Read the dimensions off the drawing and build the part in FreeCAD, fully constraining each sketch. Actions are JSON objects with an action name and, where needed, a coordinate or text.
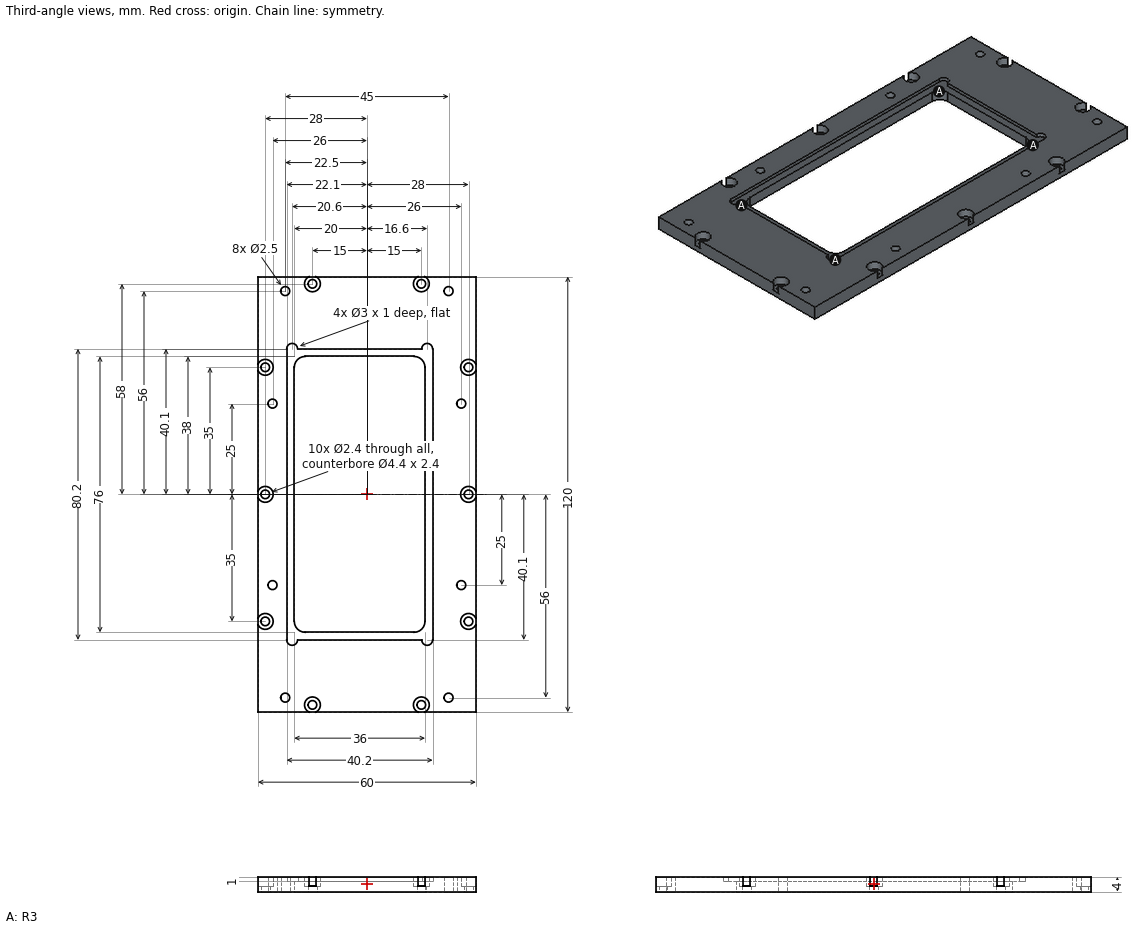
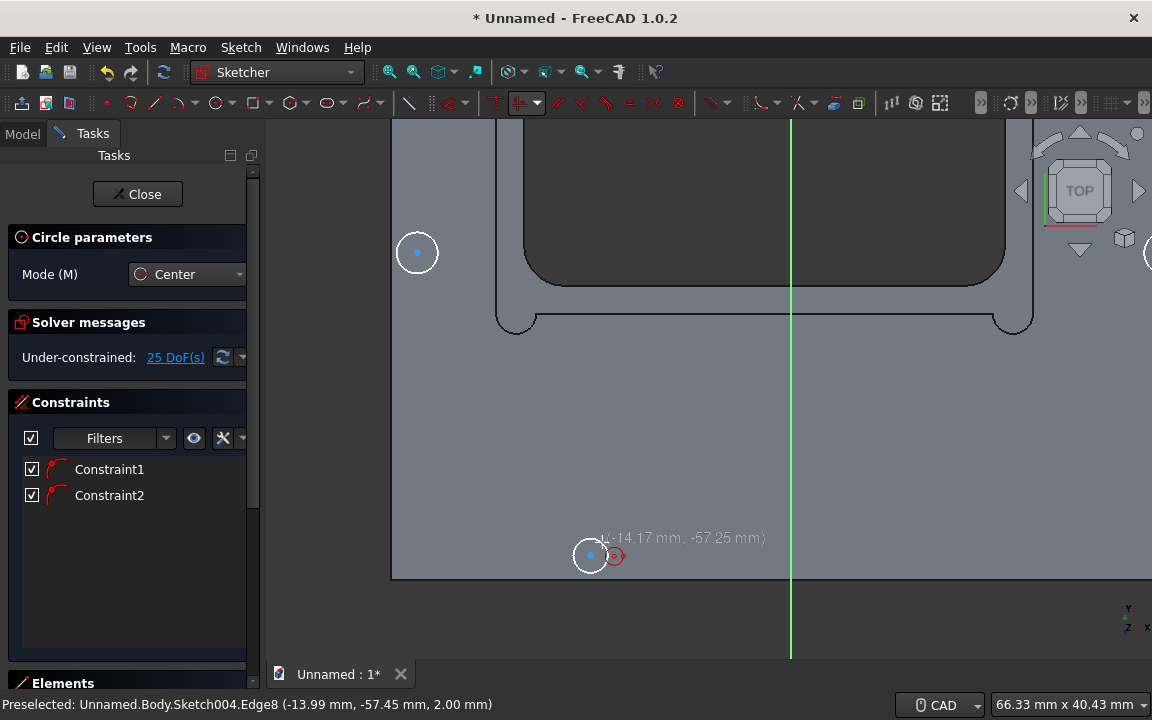
{"action": "scroll", "coordinate": [602, 543], "scroll_direction": "down", "scroll_amount": 8}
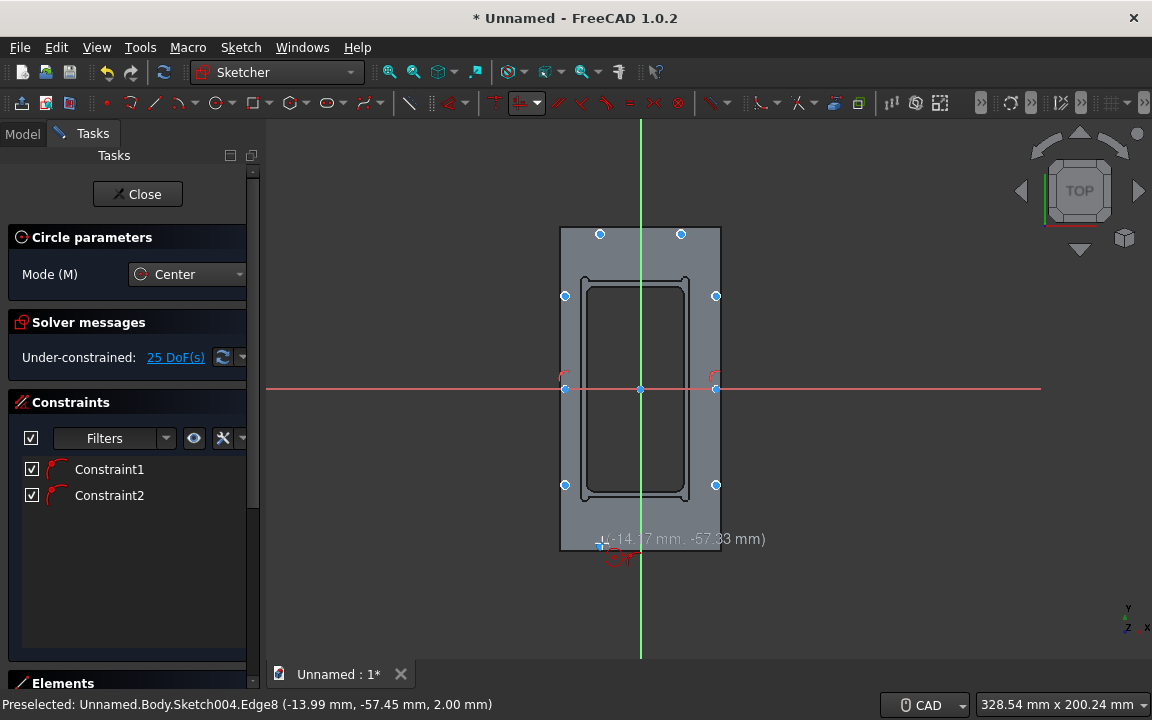
{"action": "scroll", "coordinate": [681, 546], "scroll_direction": "up", "scroll_amount": 10}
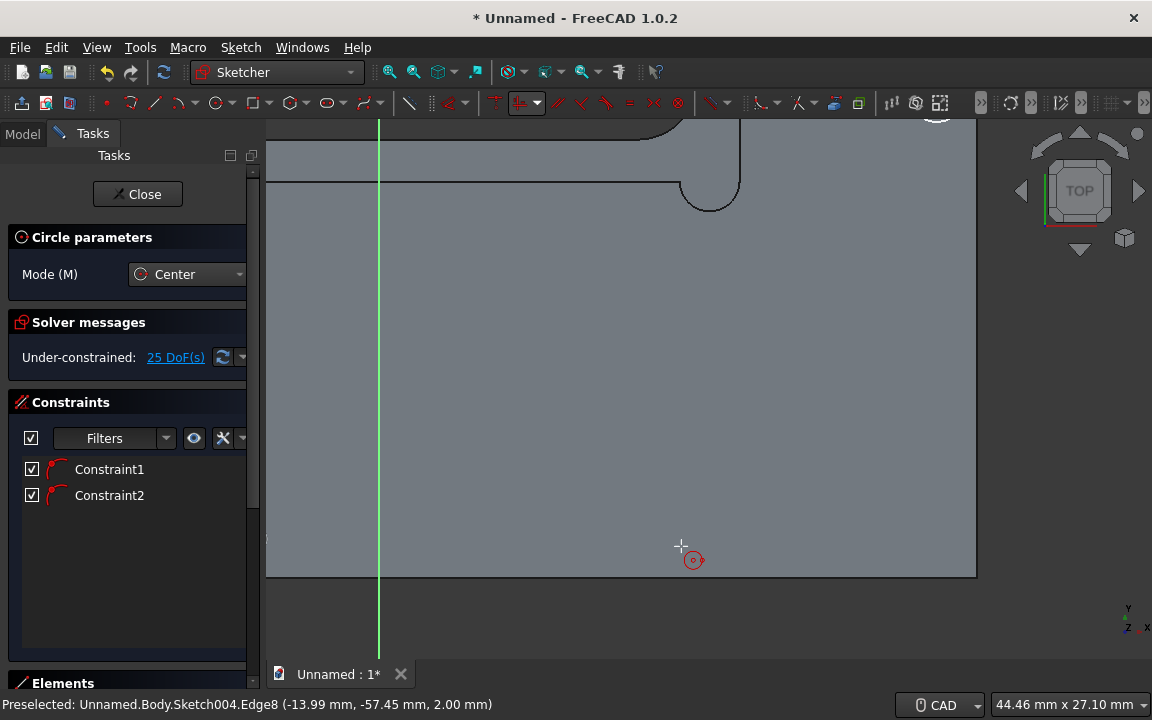
{"action": "scroll", "coordinate": [681, 547], "scroll_direction": "down", "scroll_amount": 10}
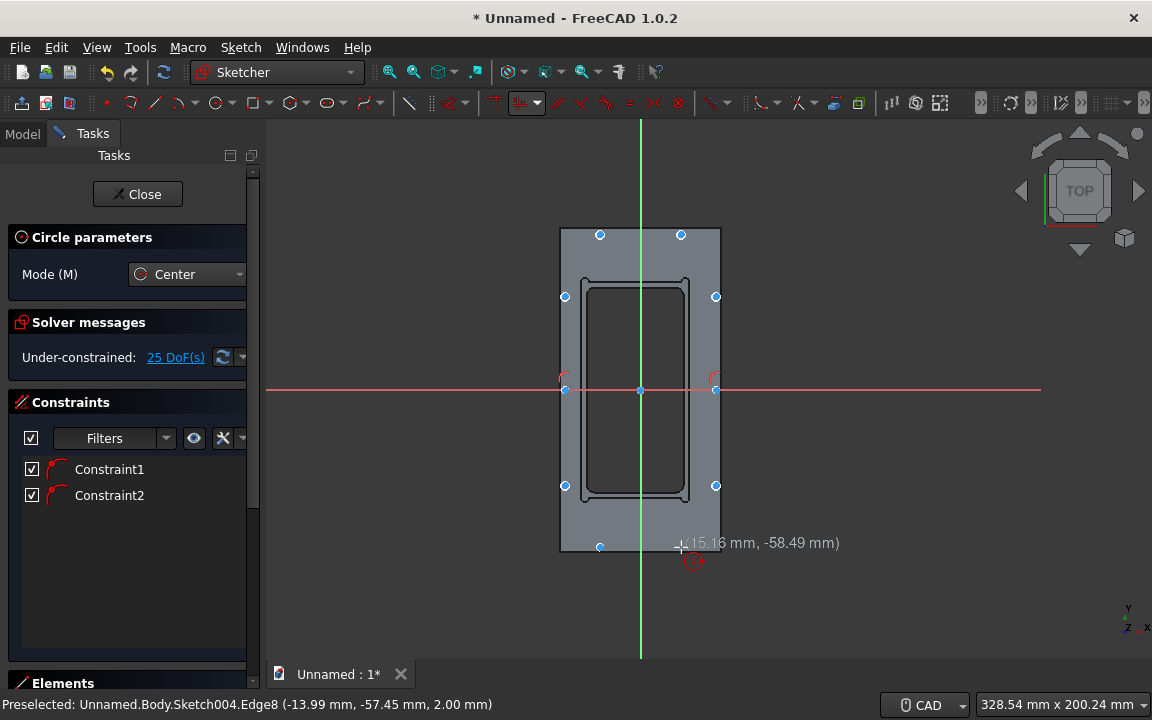
{"action": "left_click", "coordinate": [681, 547]}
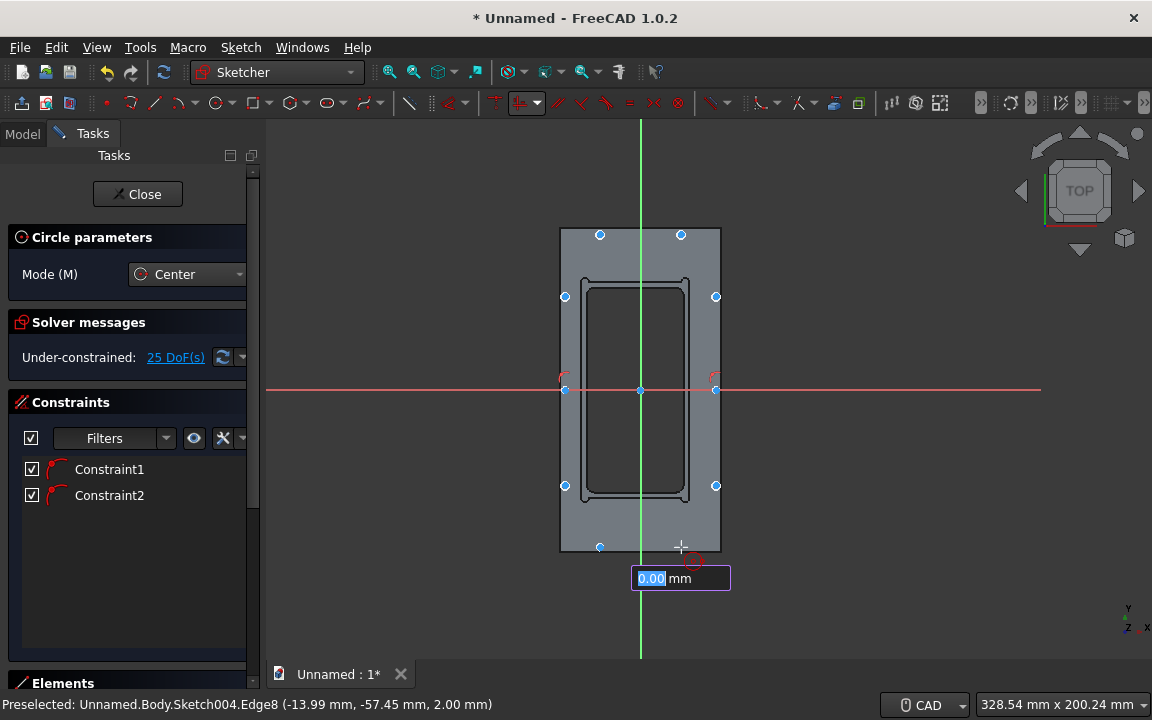
{"action": "scroll", "coordinate": [683, 544], "scroll_direction": "up", "scroll_amount": 8}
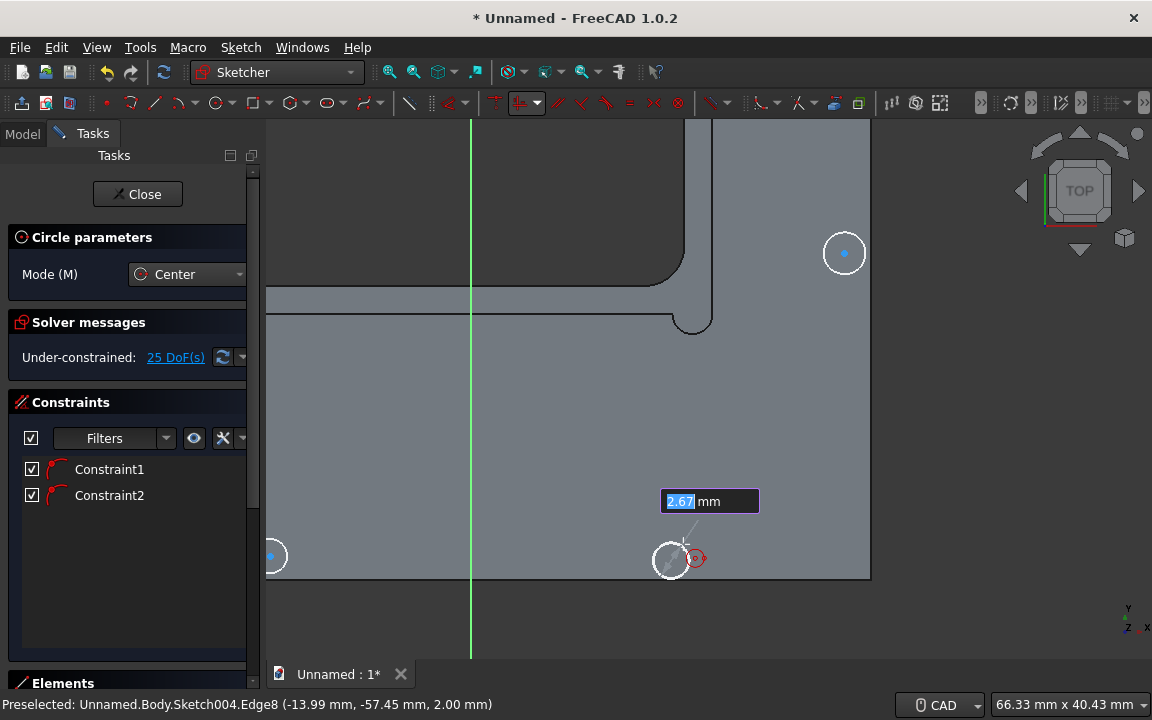
{"action": "left_click", "coordinate": [682, 542]}
{"action": "key", "text": "Escape"}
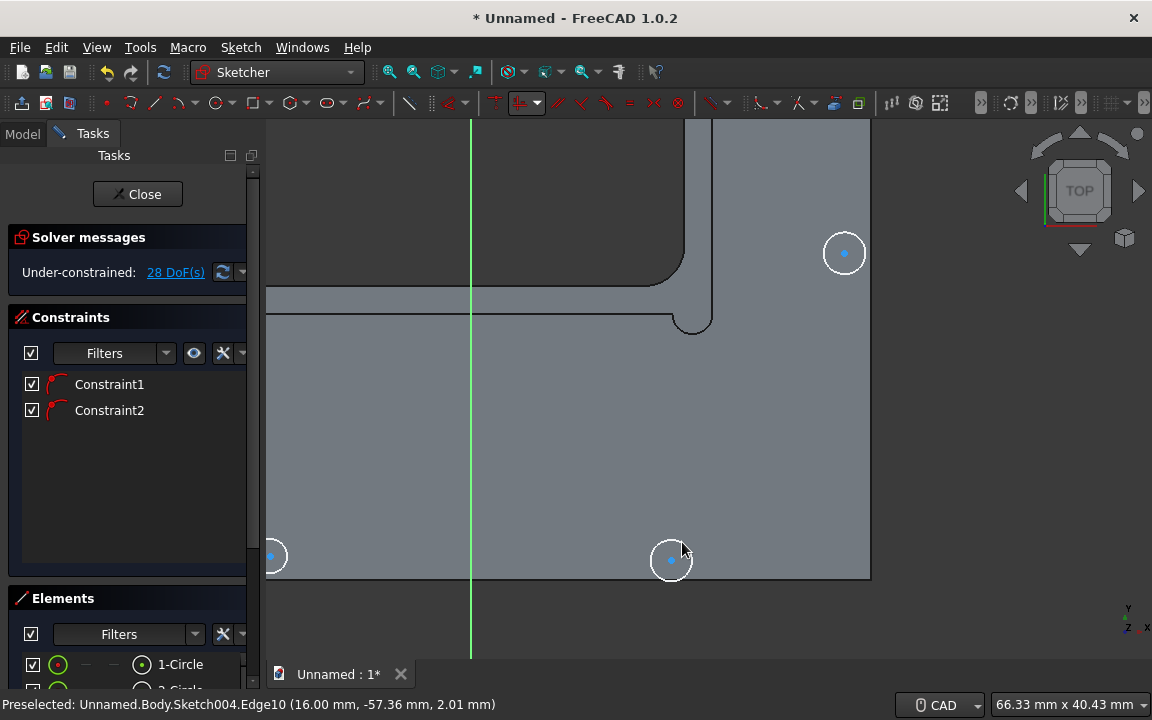
{"action": "scroll", "coordinate": [683, 543], "scroll_direction": "down", "scroll_amount": 8}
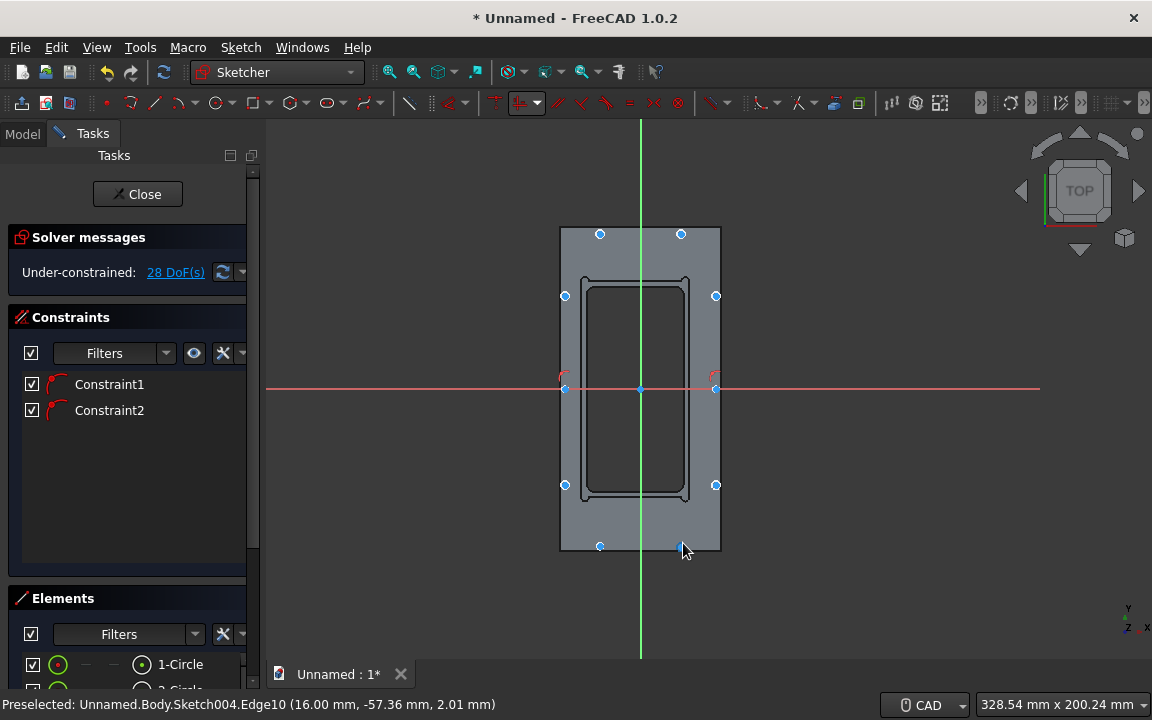
{"action": "scroll", "coordinate": [567, 387], "scroll_direction": "up", "scroll_amount": 10}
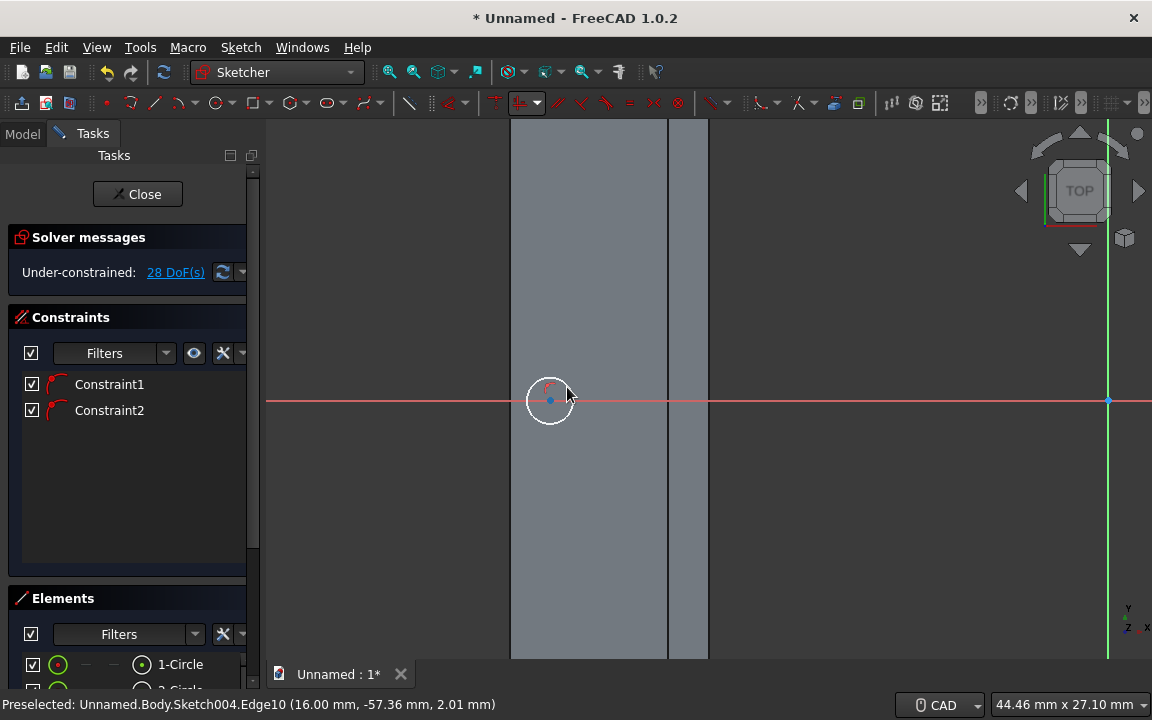
{"action": "left_click", "coordinate": [566, 384]}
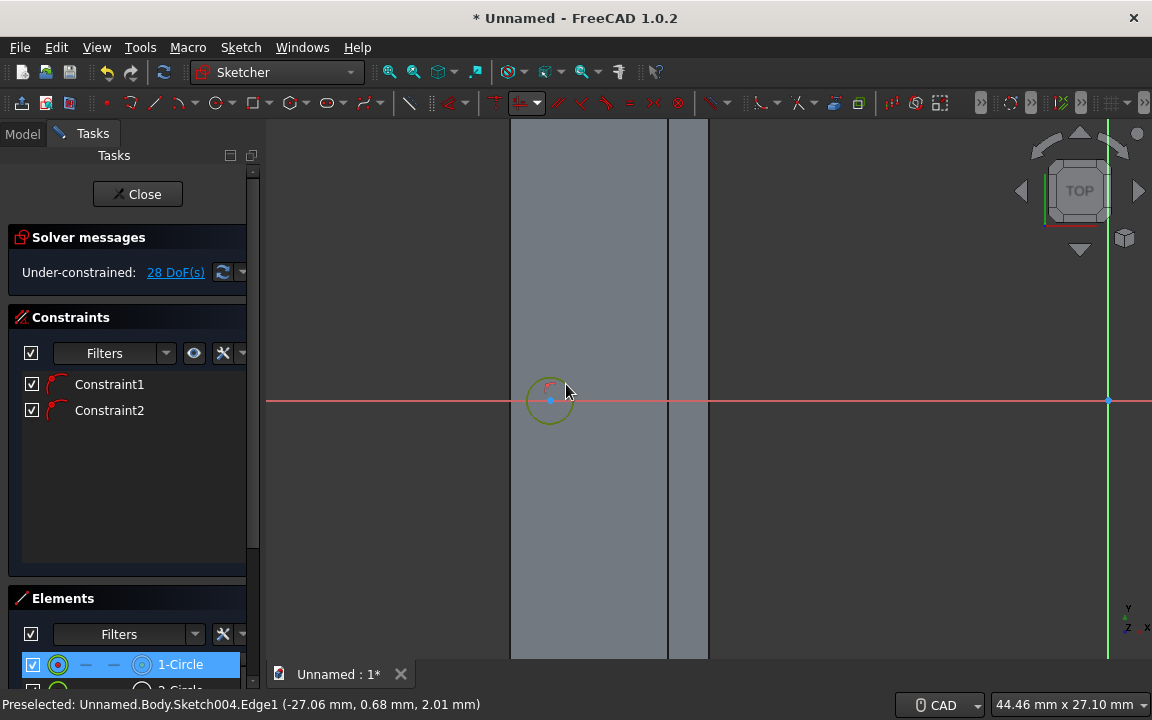
{"action": "scroll", "coordinate": [567, 387], "scroll_direction": "down", "scroll_amount": 10}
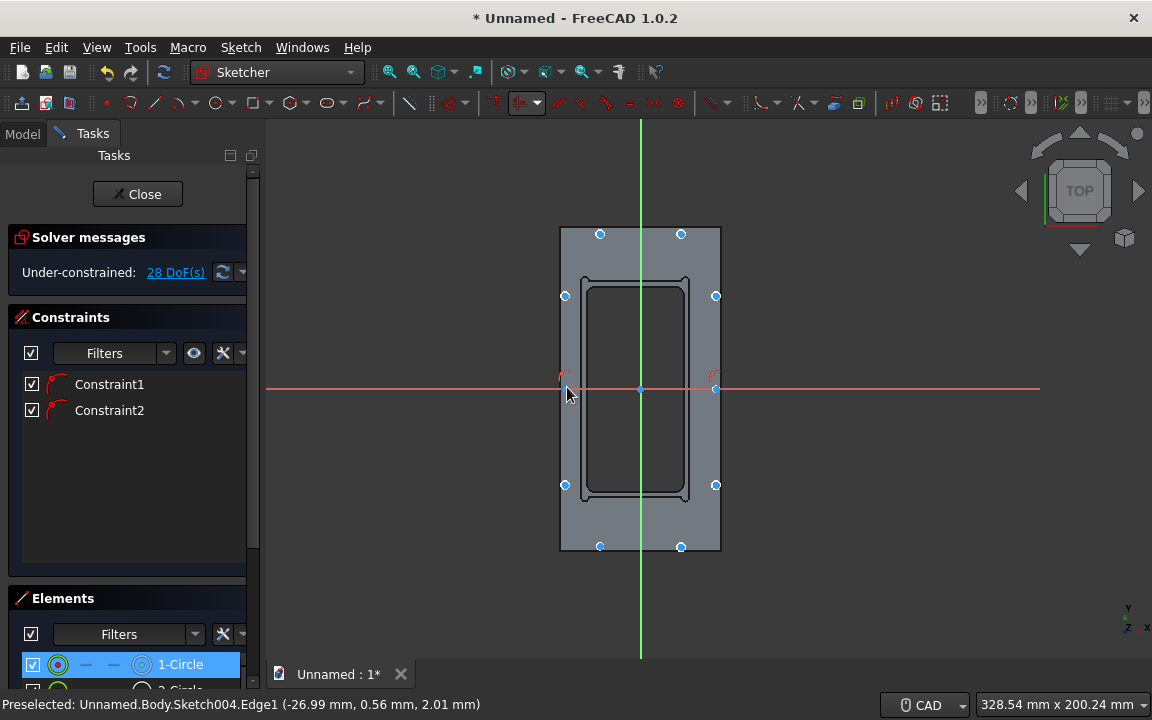
{"action": "scroll", "coordinate": [718, 387], "scroll_direction": "up", "scroll_amount": 10}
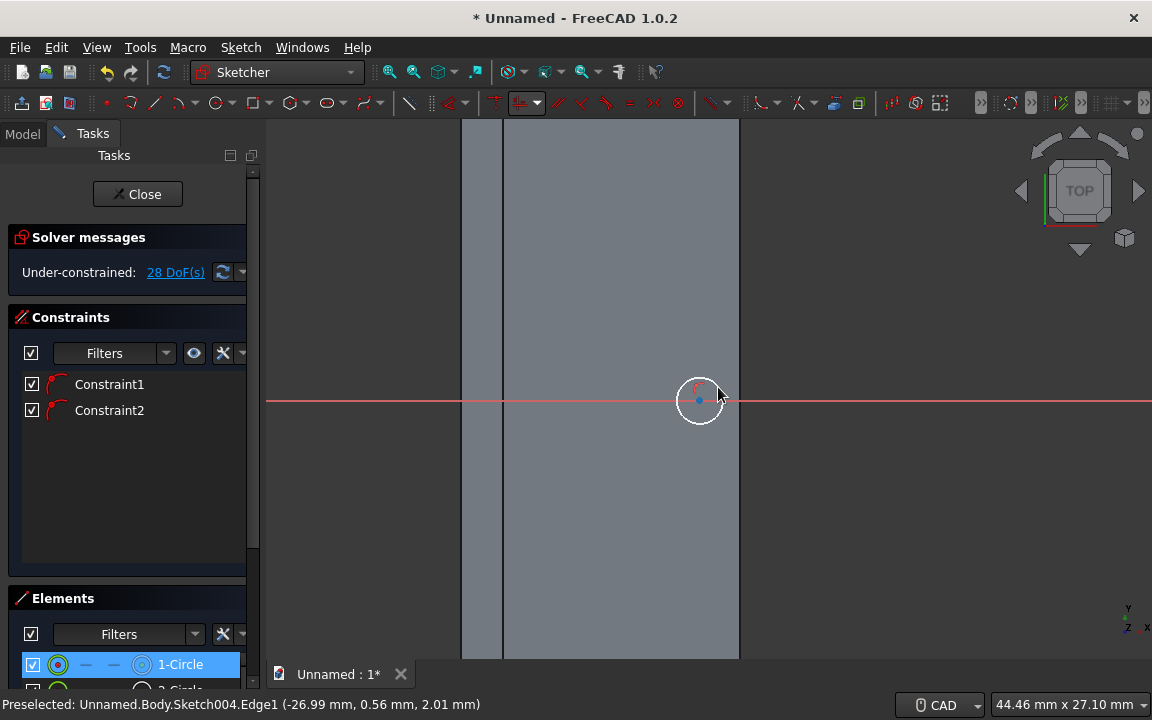
{"action": "left_click", "coordinate": [716, 384]}